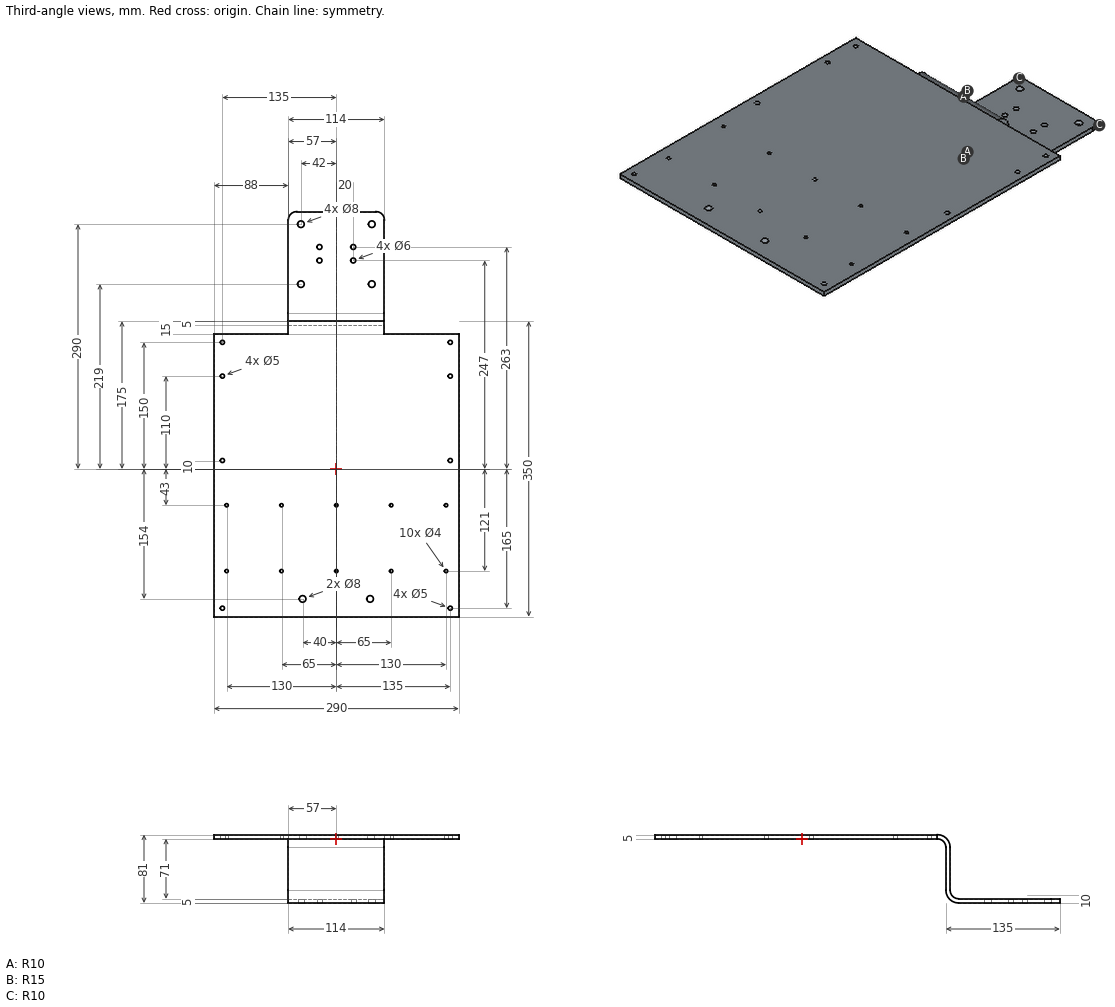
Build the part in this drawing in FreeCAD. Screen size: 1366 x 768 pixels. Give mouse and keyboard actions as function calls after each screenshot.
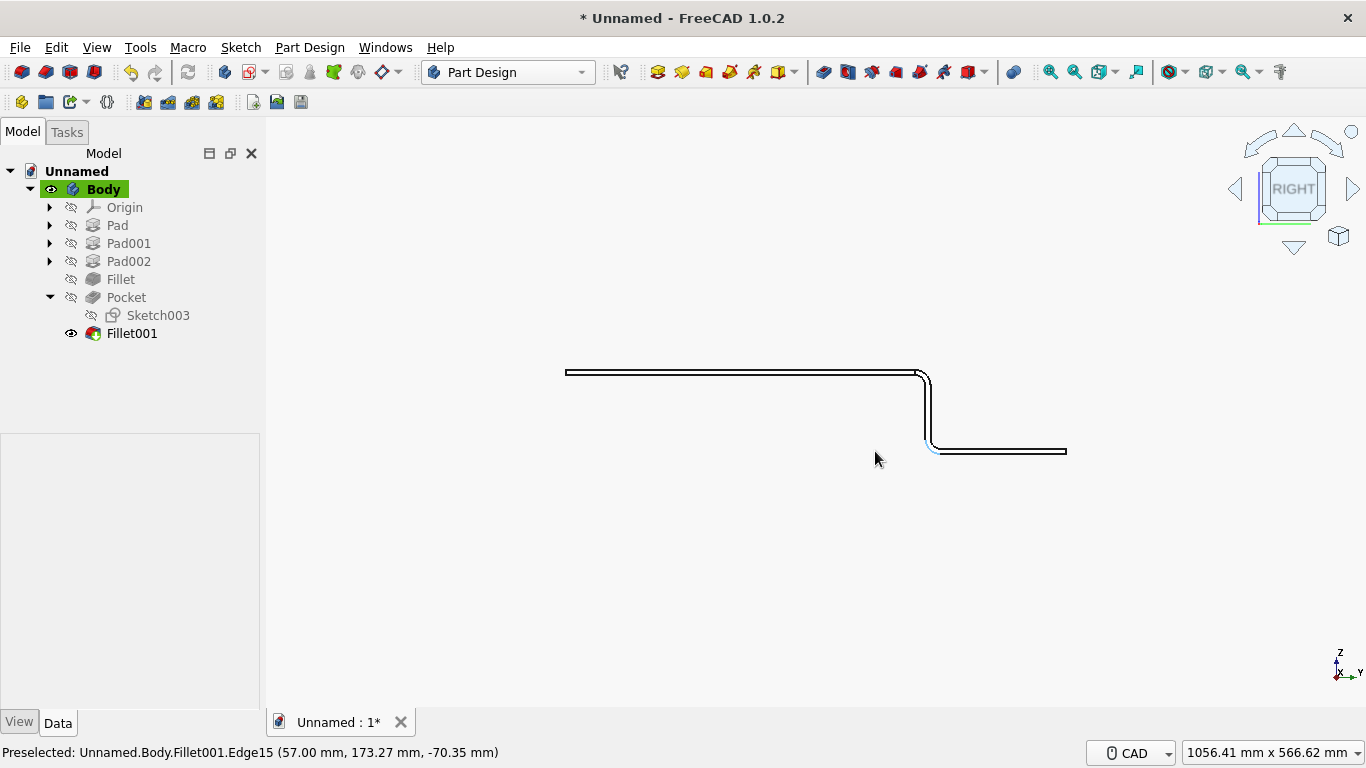
scroll(1066, 451, up, 11)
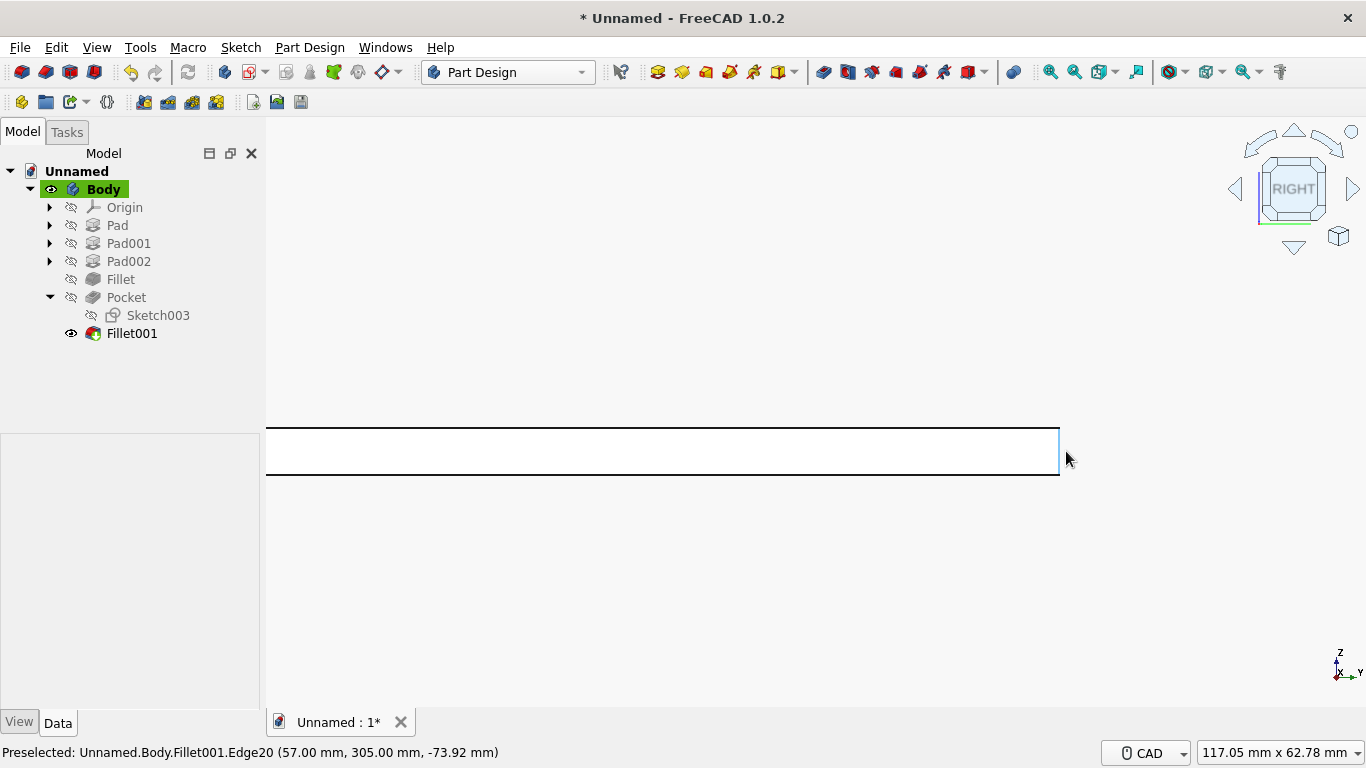
click(1059, 451)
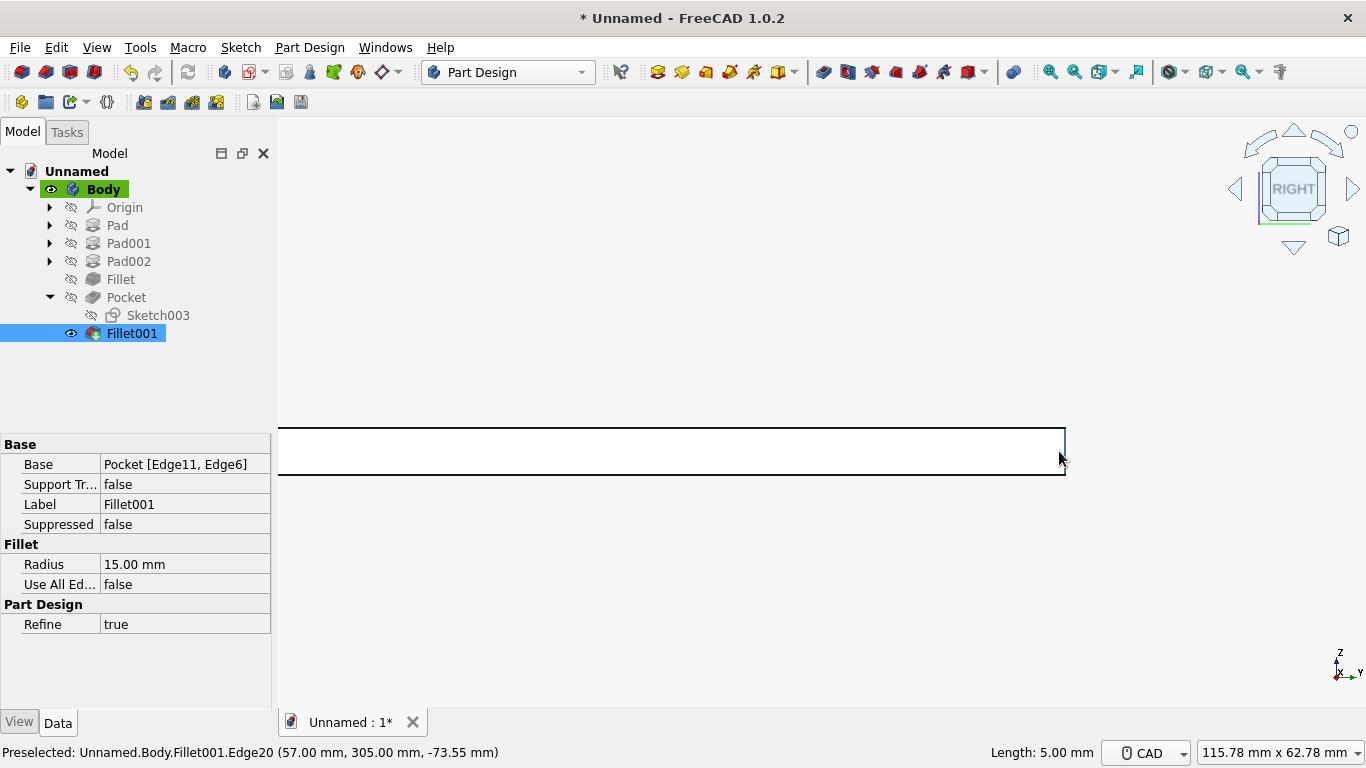
key(v)
key(f)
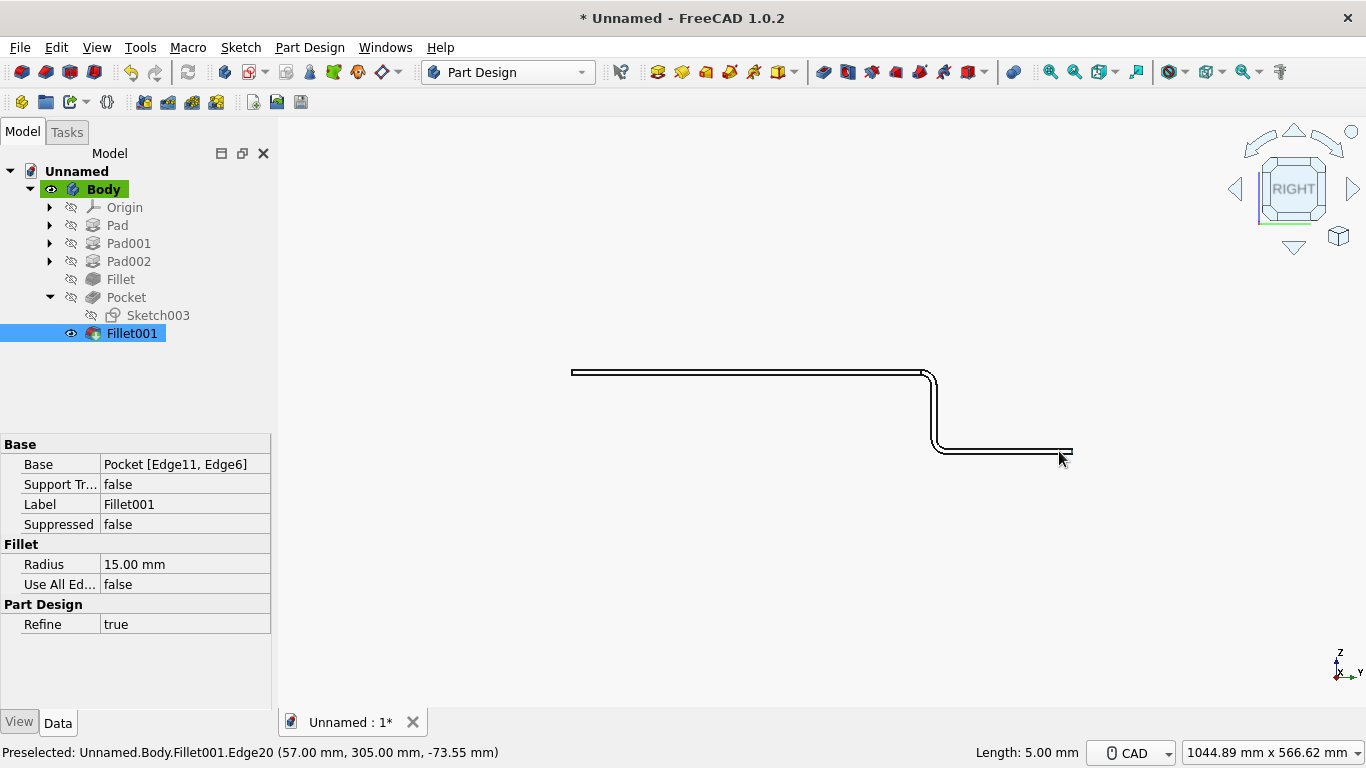
key(5)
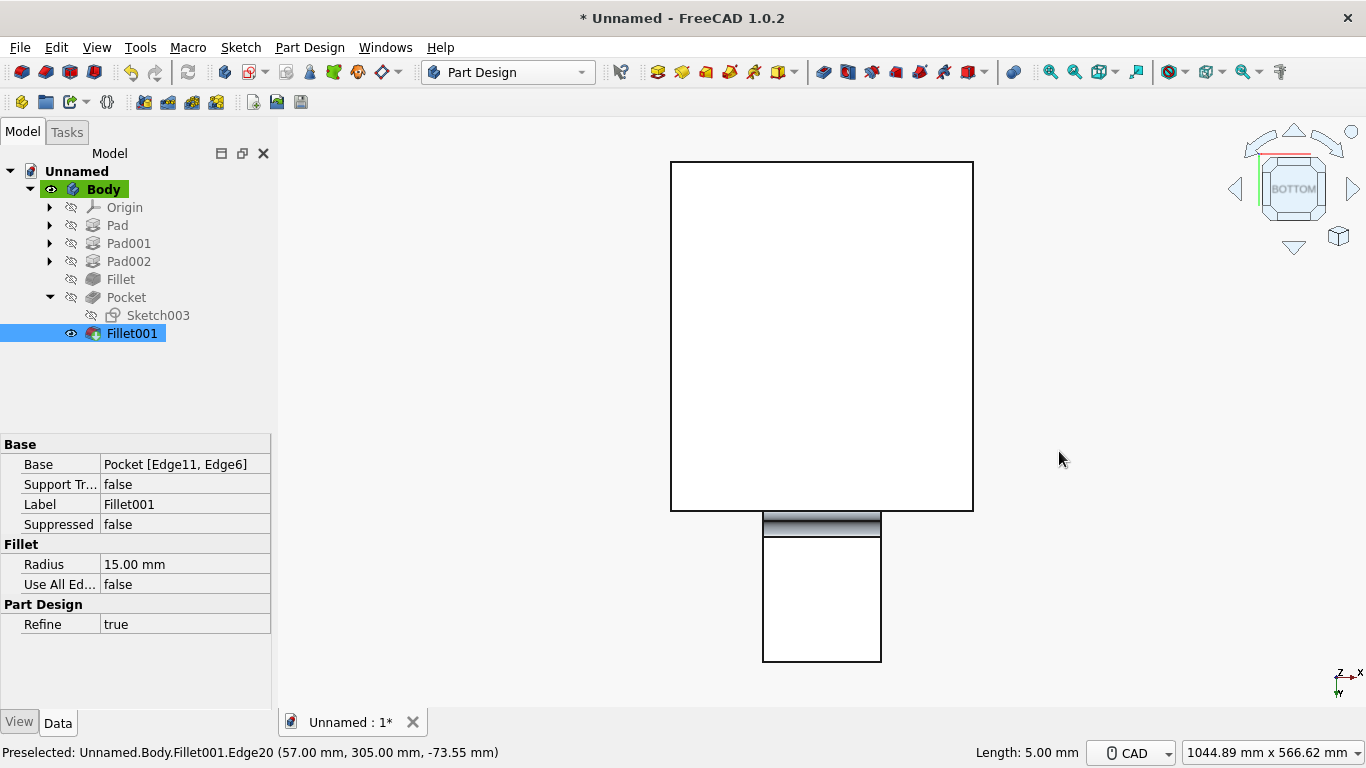
scroll(763, 661, up, 11)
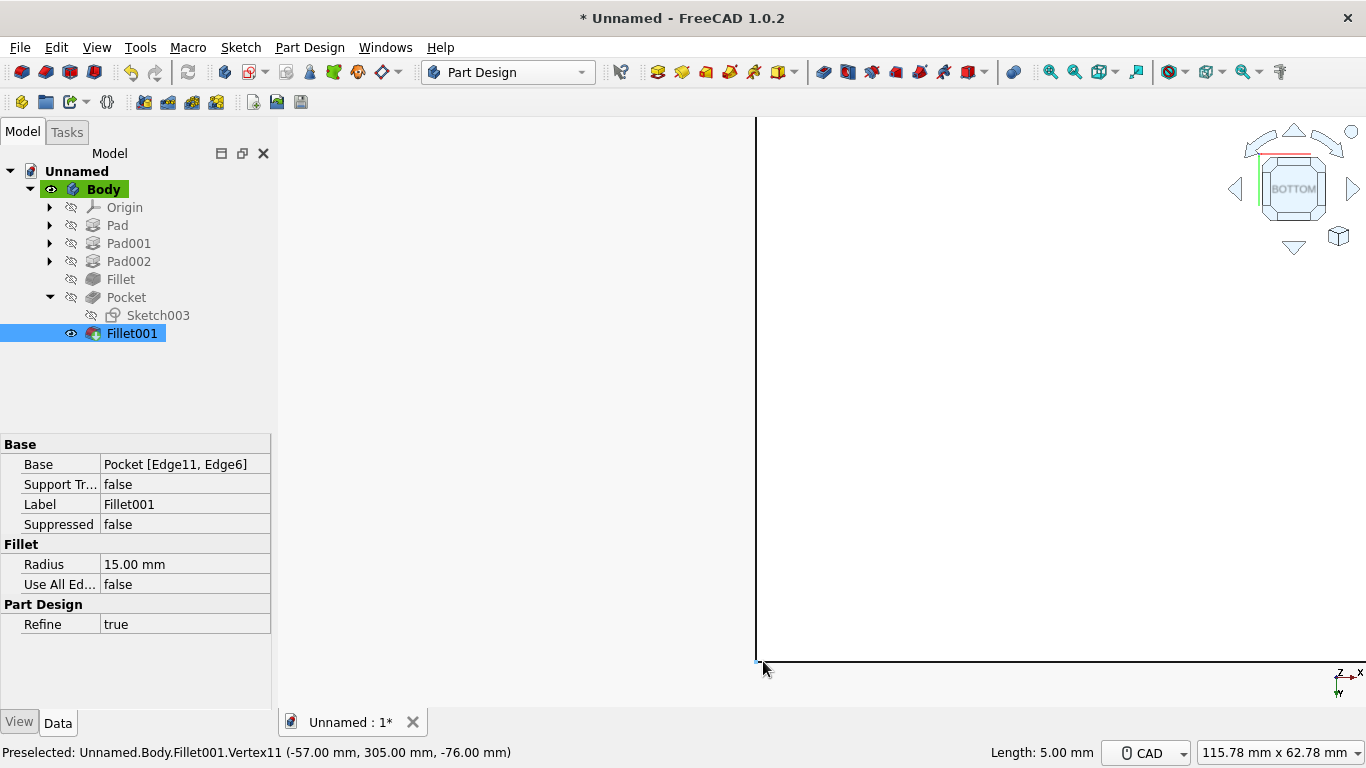
click(1052, 72)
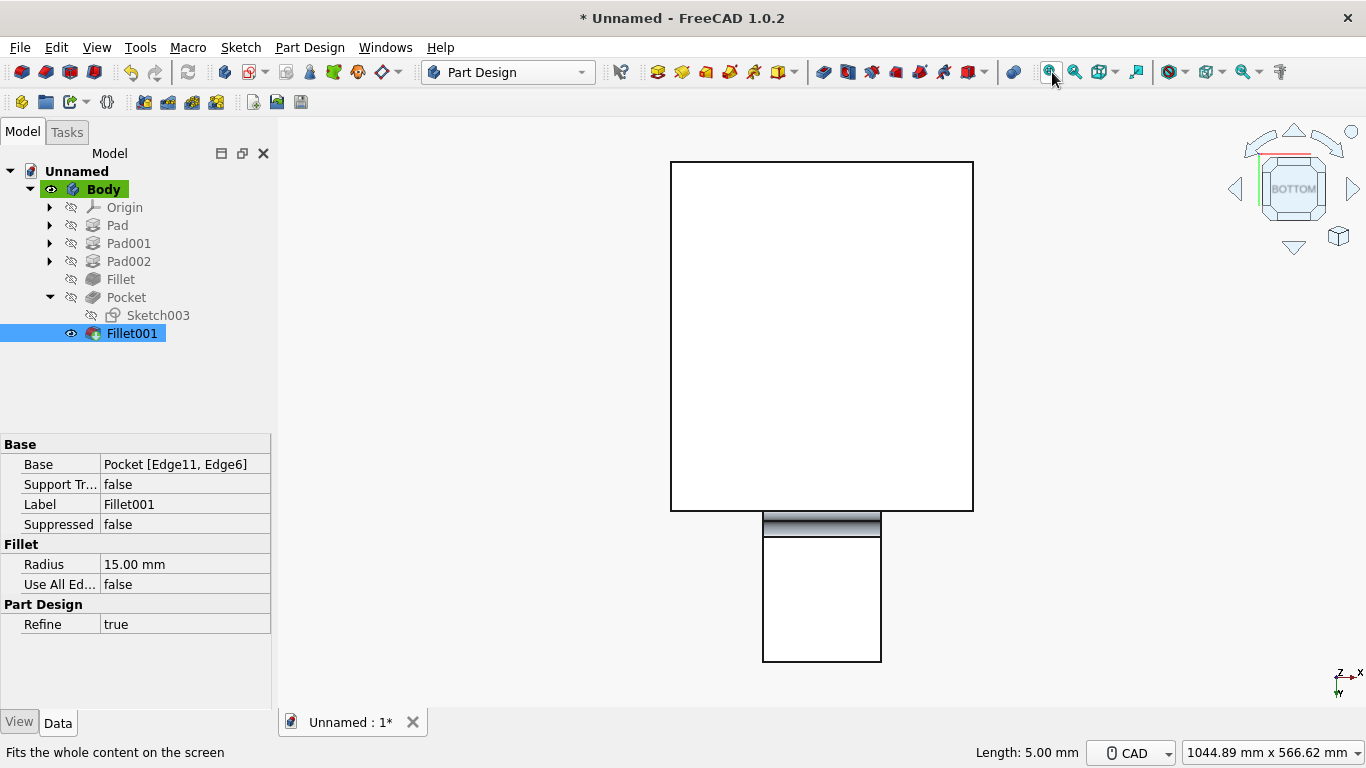
key(4)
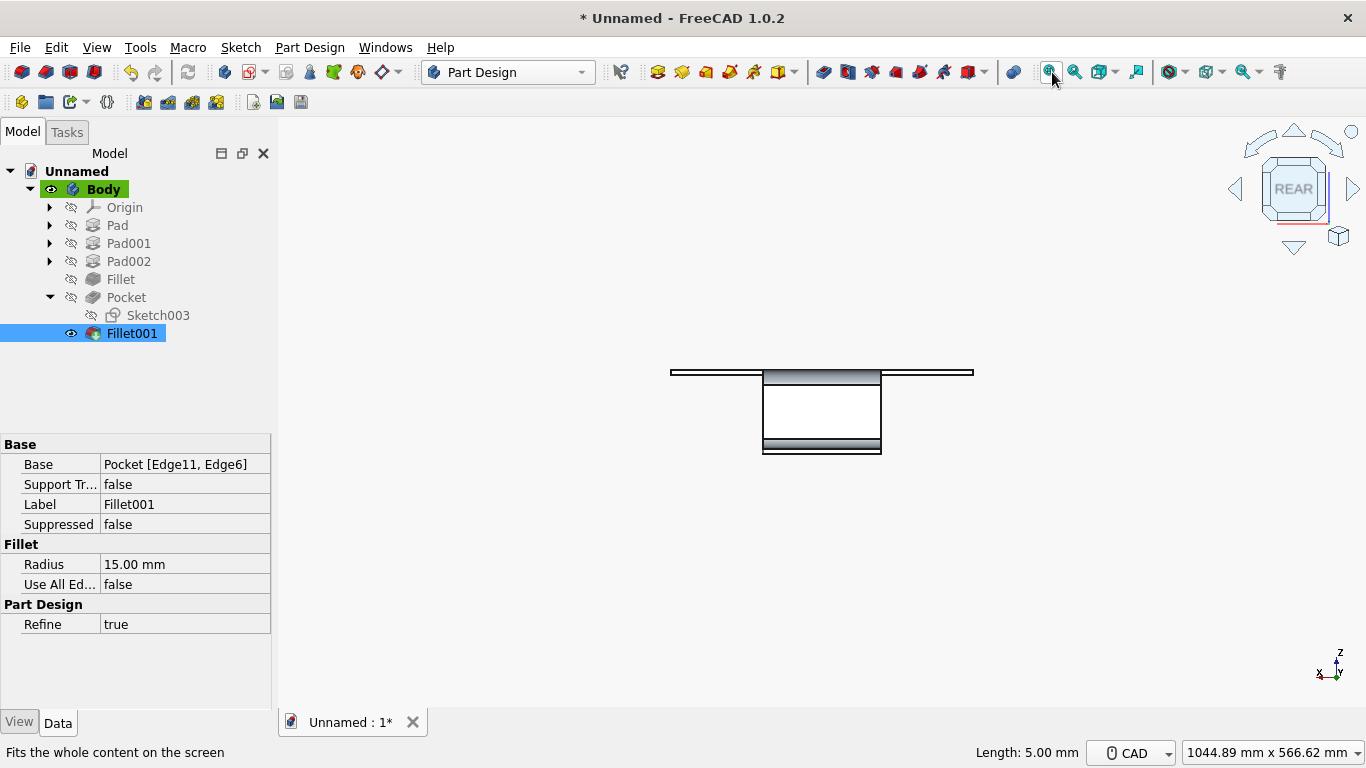
click(1052, 72)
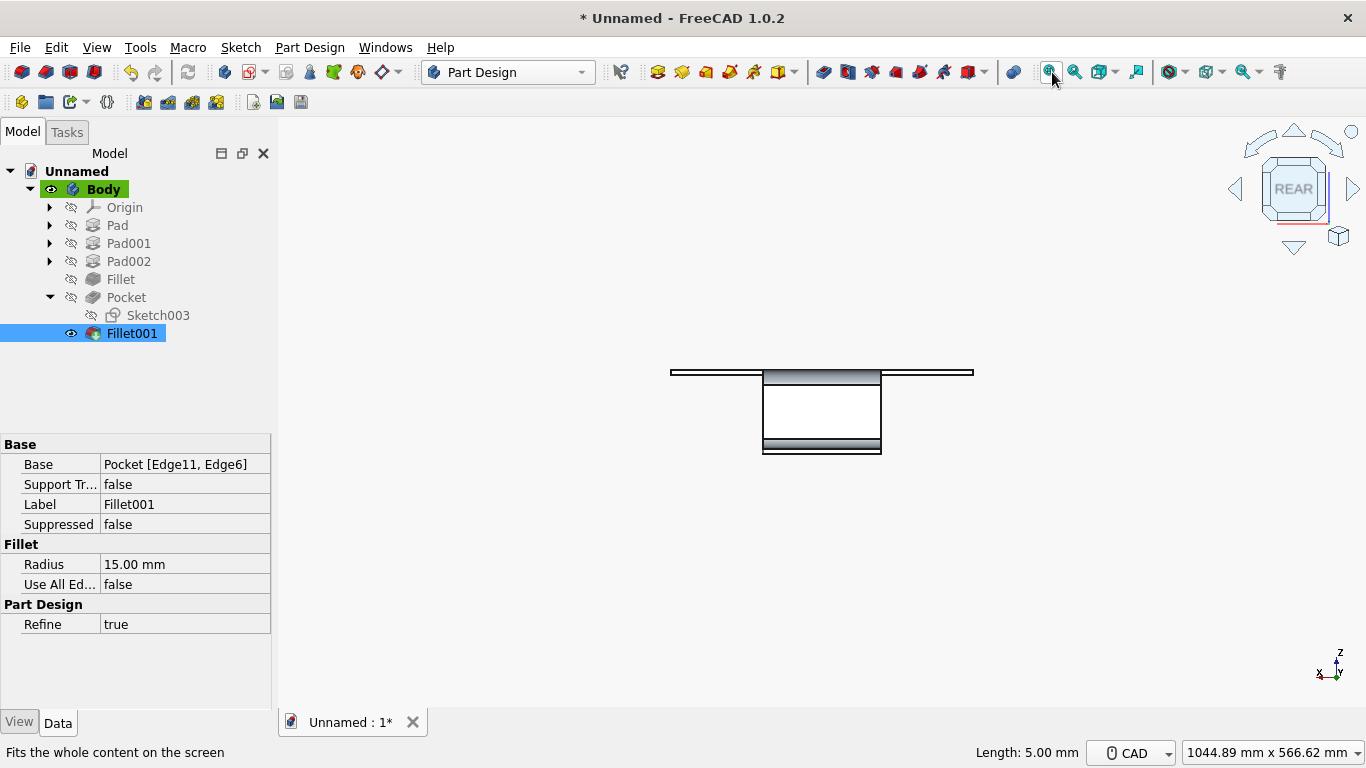
scroll(881, 451, up, 11)